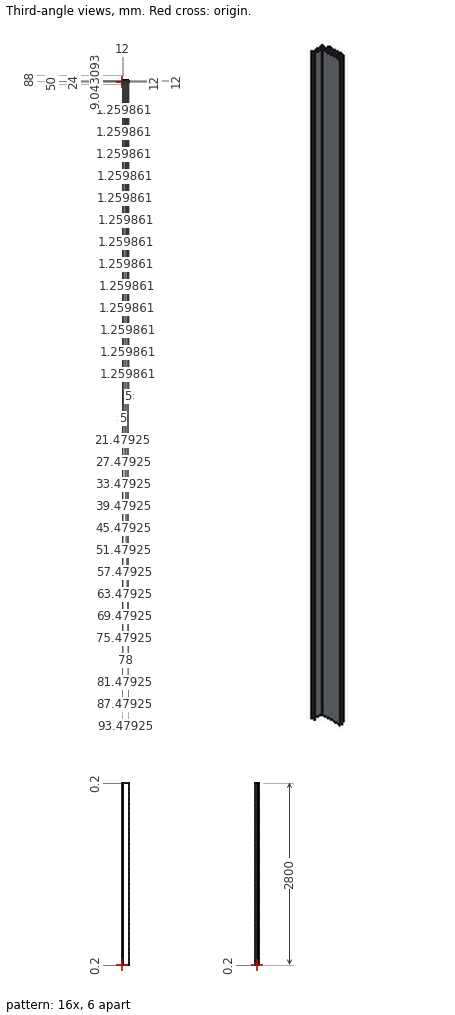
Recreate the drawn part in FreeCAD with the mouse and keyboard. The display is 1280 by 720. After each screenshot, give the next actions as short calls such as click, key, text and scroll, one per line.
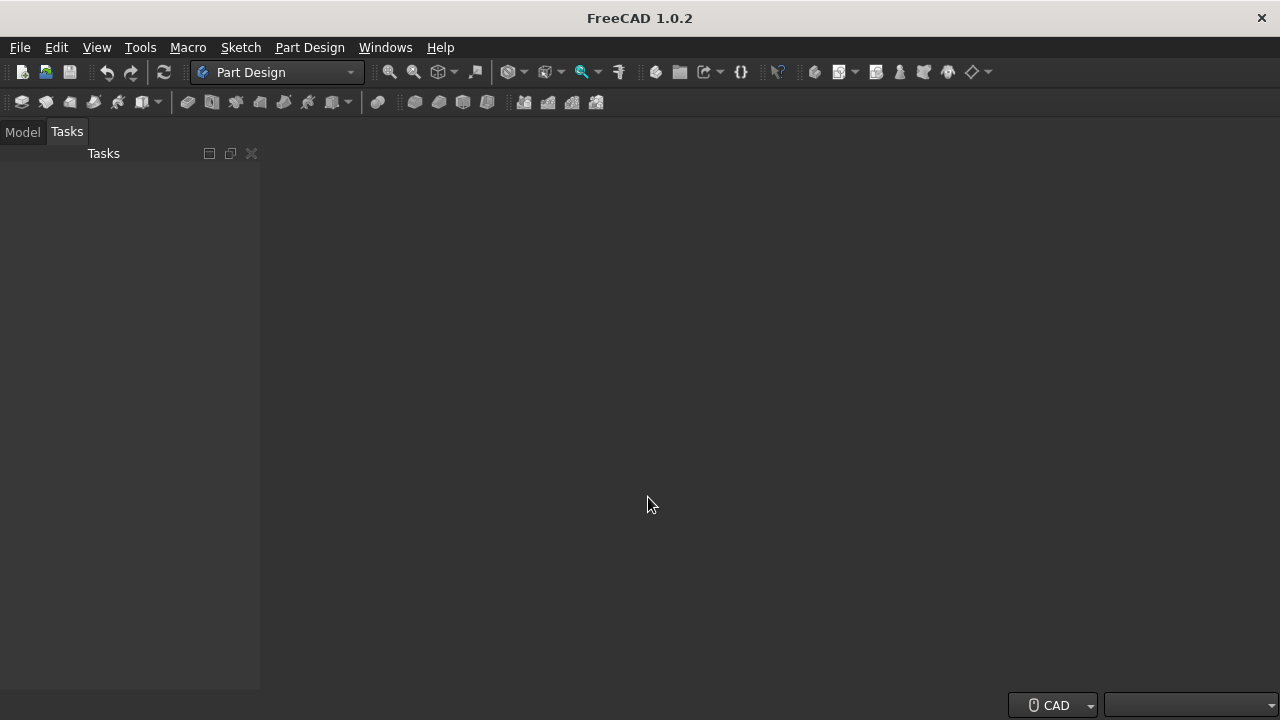
click(22, 72)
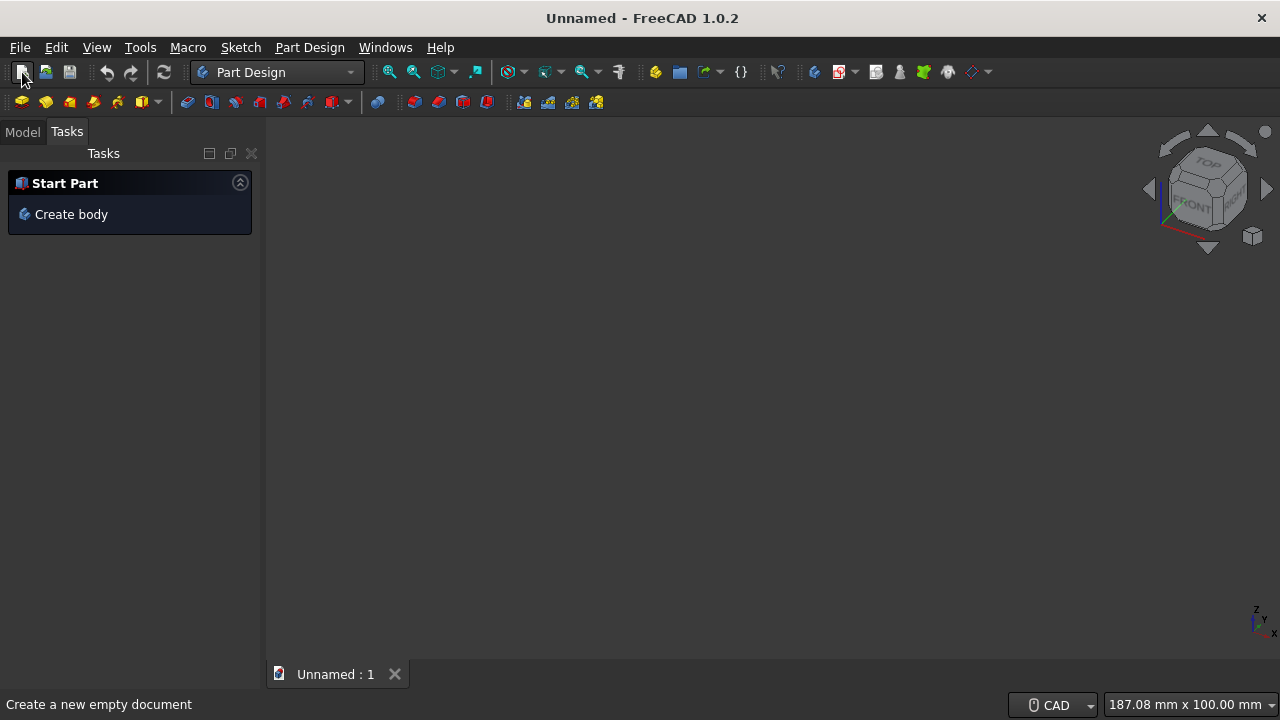
click(840, 72)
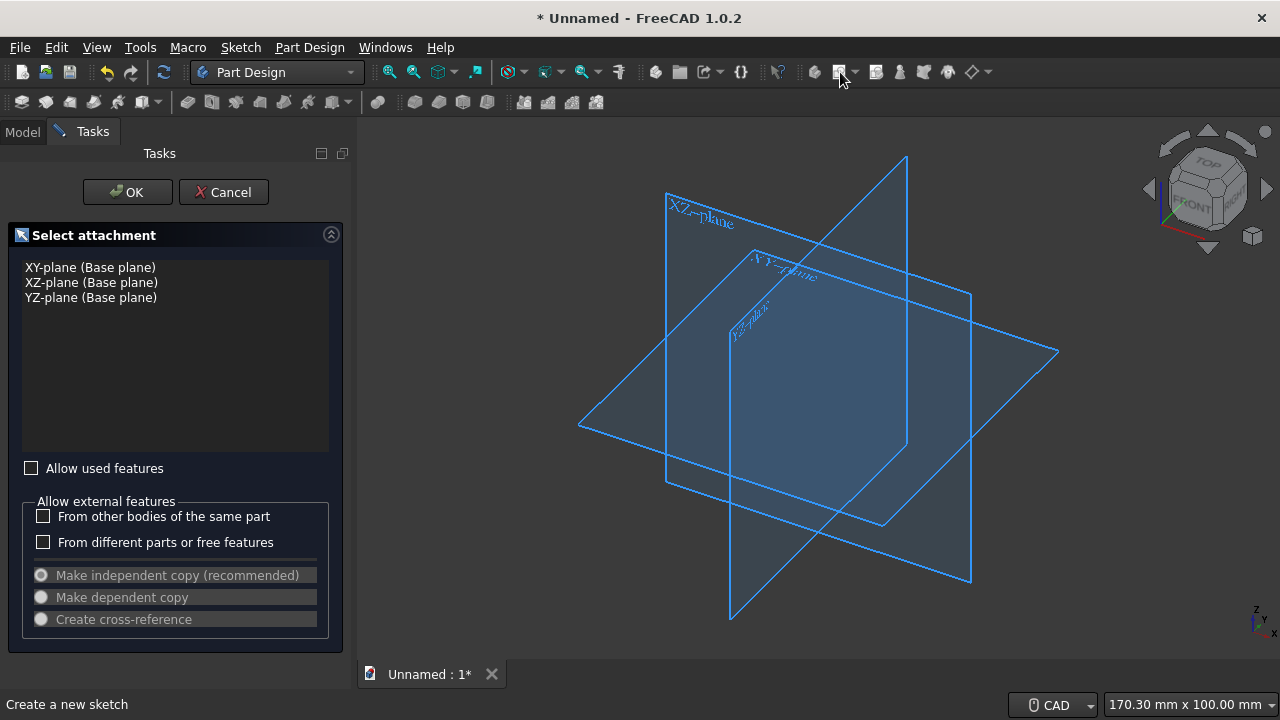
click(82, 268)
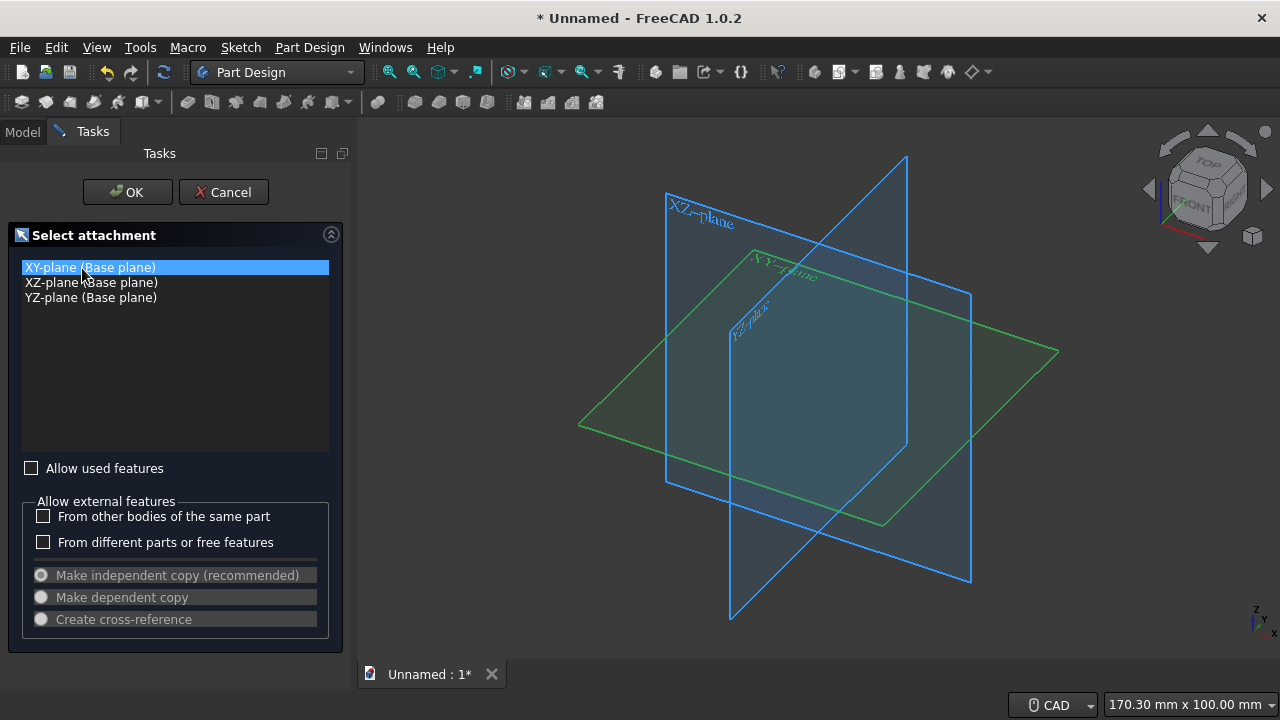
click(128, 192)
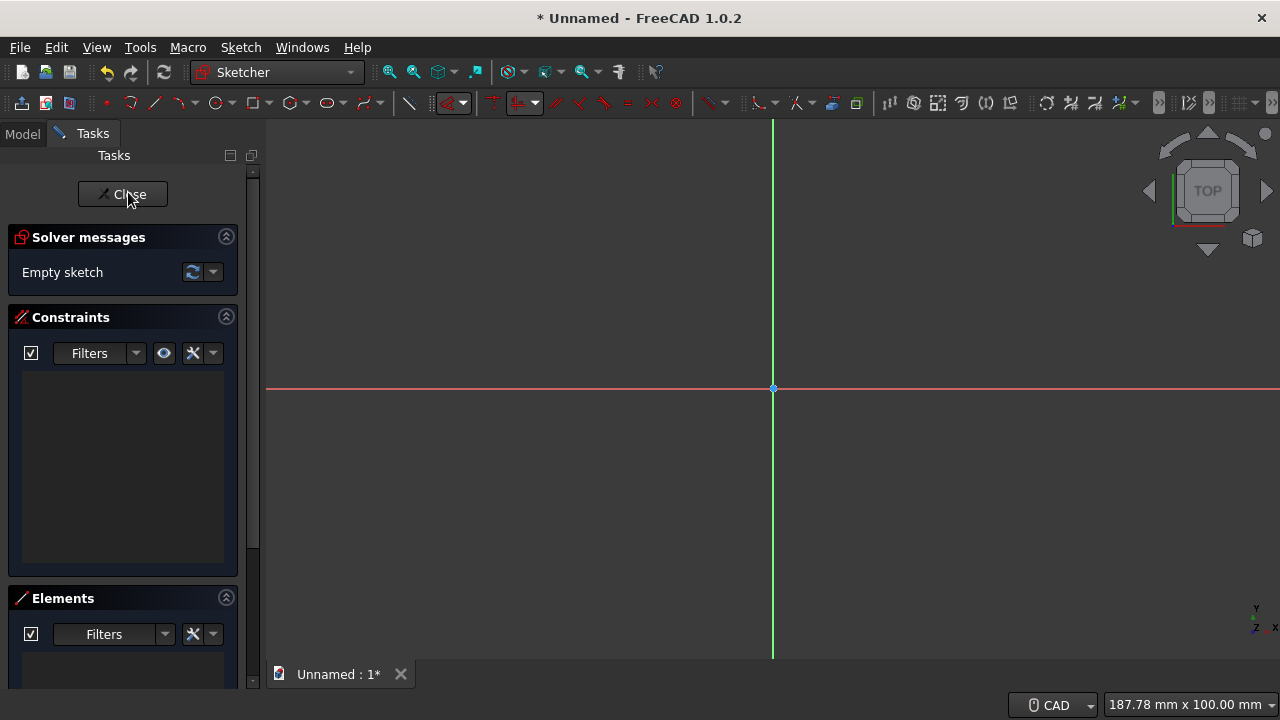
scroll(294, 631, down, 3)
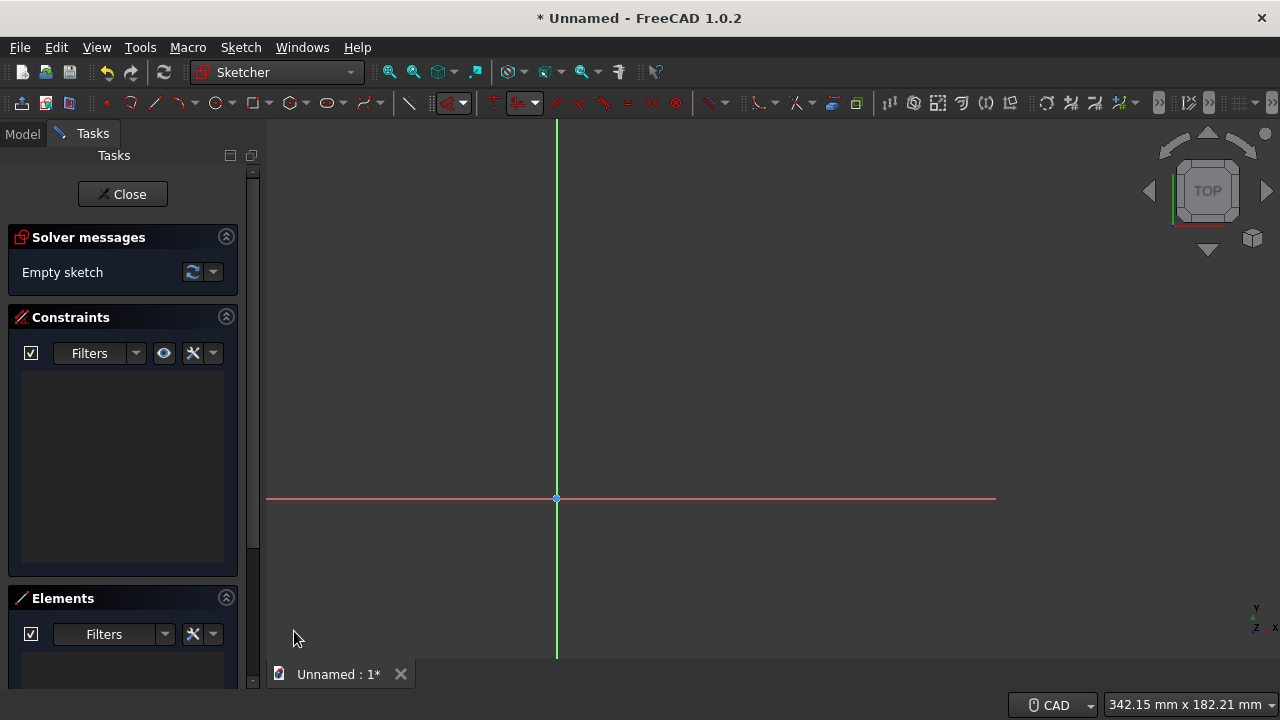
click(132, 104)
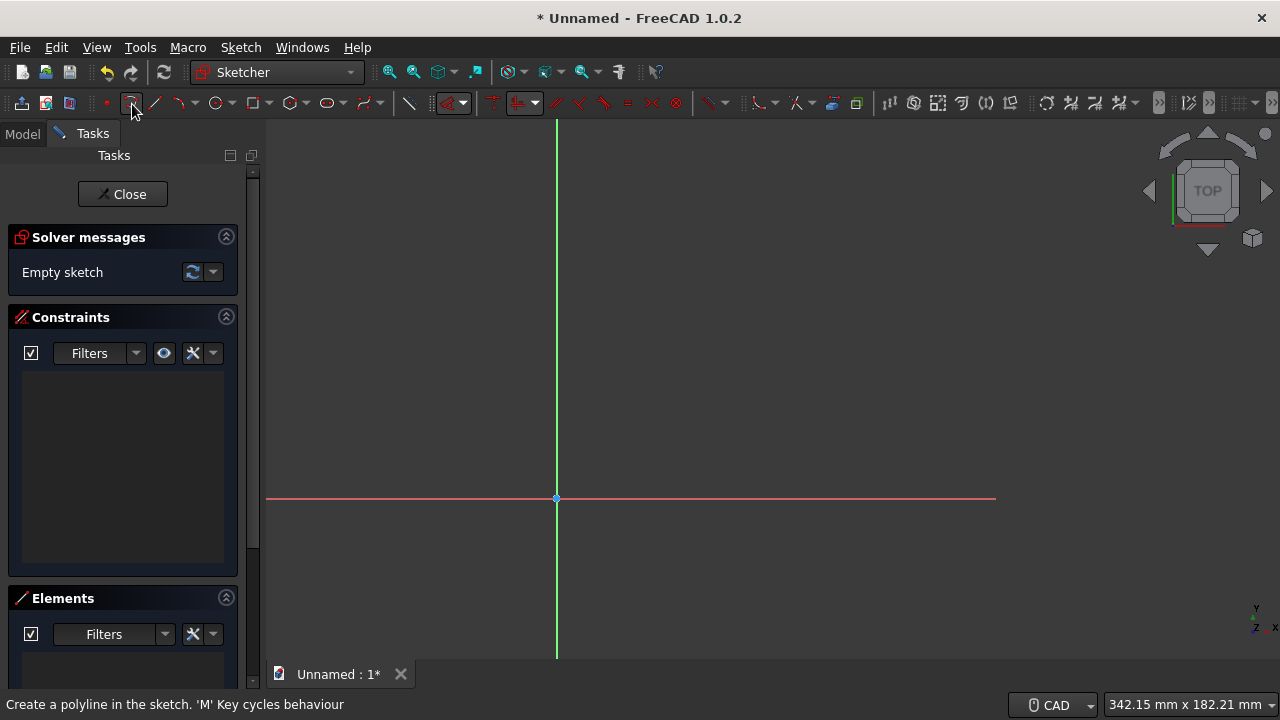
click(557, 499)
click(853, 490)
click(853, 463)
click(838, 463)
click(838, 427)
click(607, 427)
click(607, 463)
click(592, 463)
click(592, 202)
click(566, 202)
click(557, 499)
key(Escape)
key(Escape)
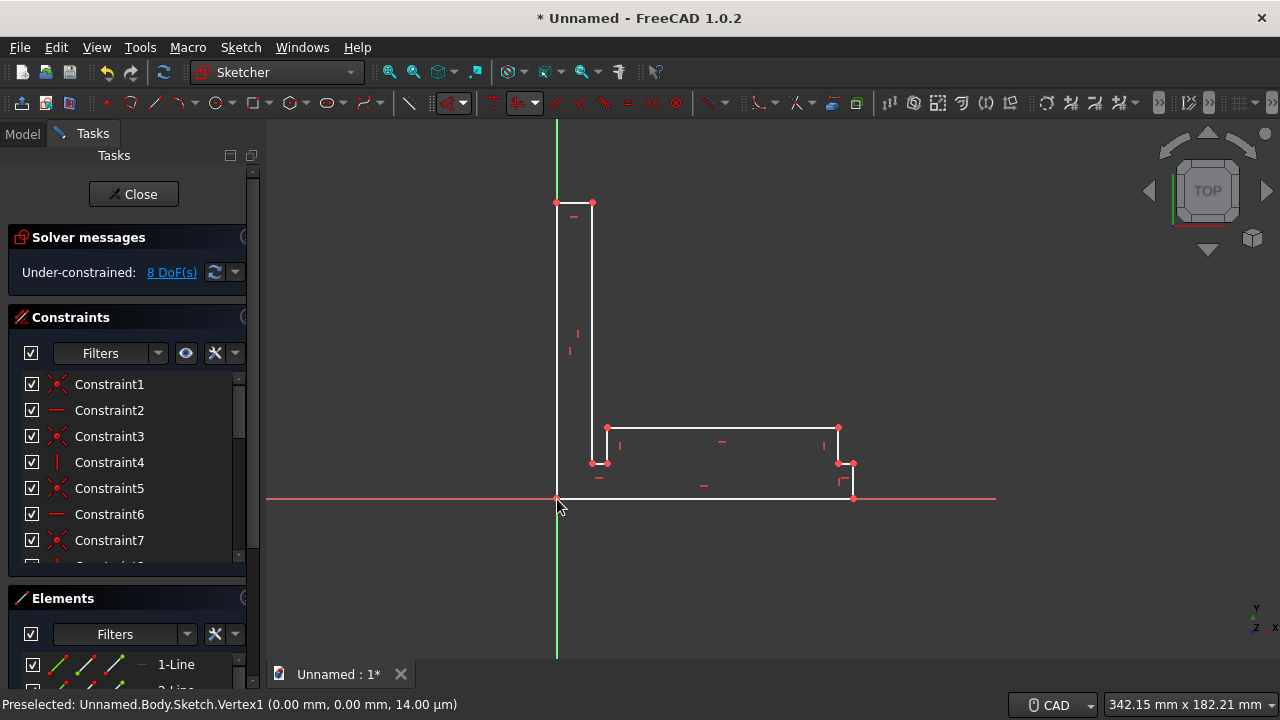
click(448, 104)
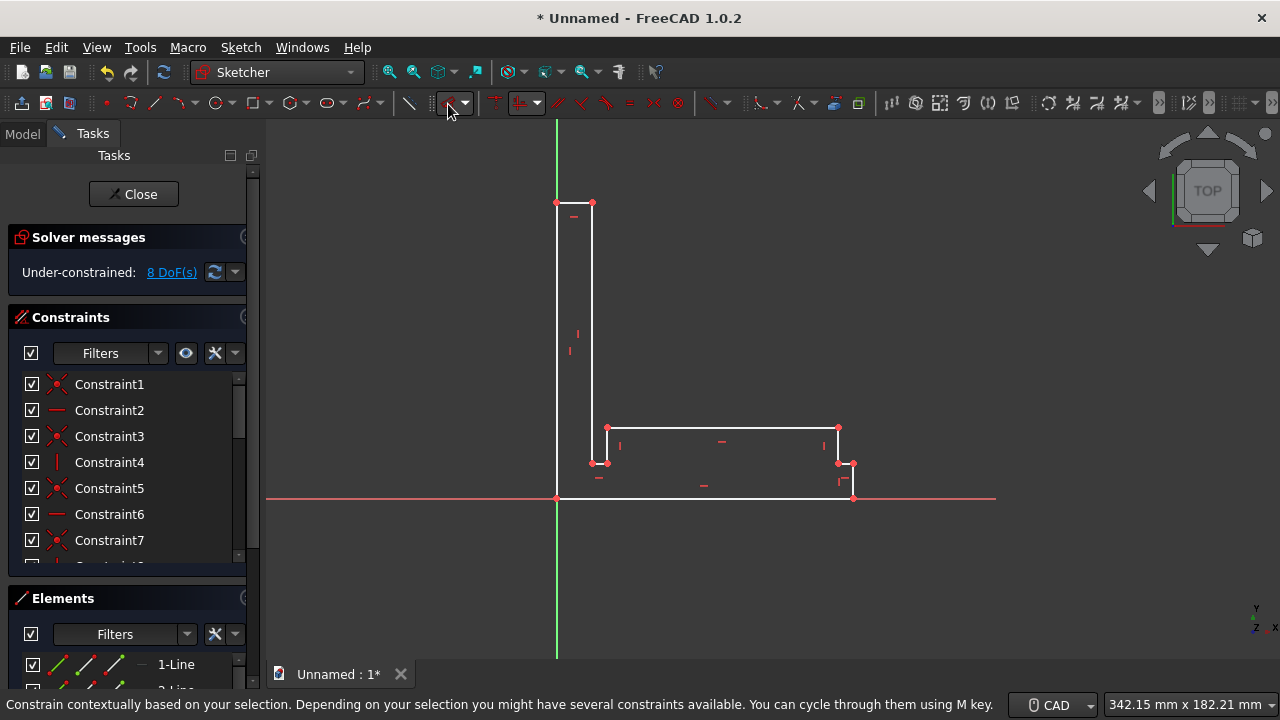
scroll(846, 464, up, 5)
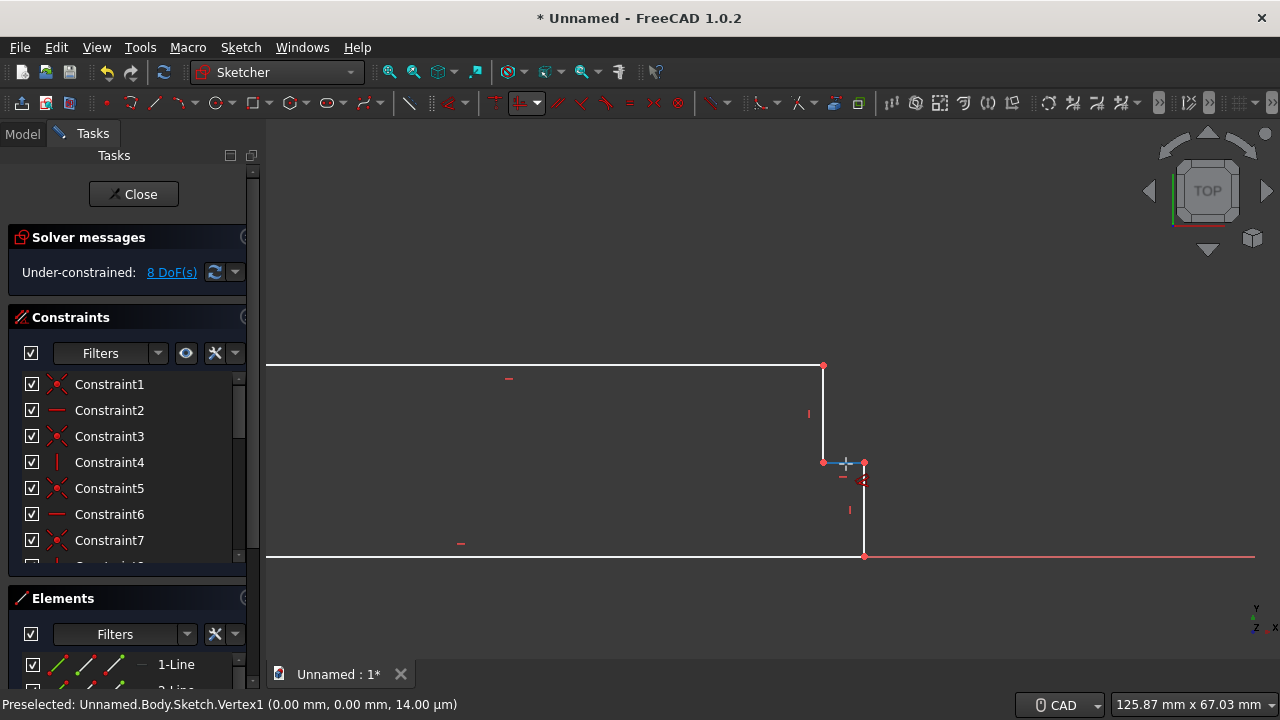
click(844, 463)
click(844, 497)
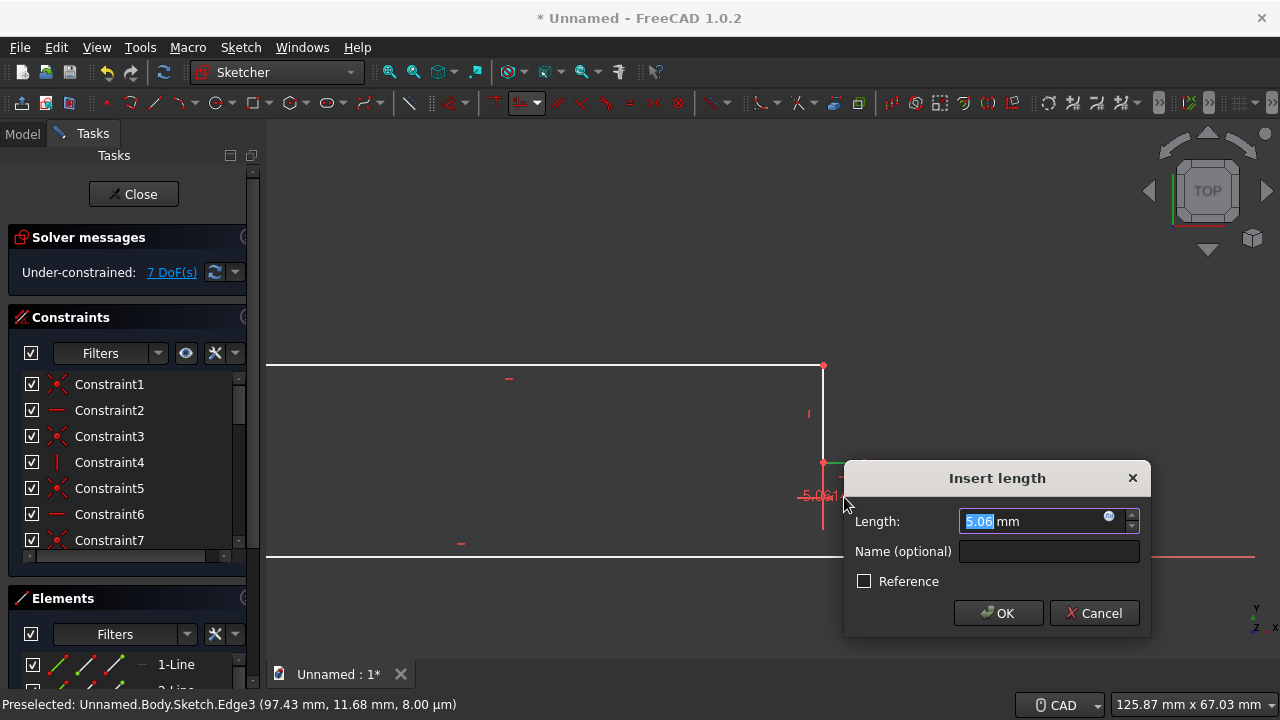
text(5)
key(Return)